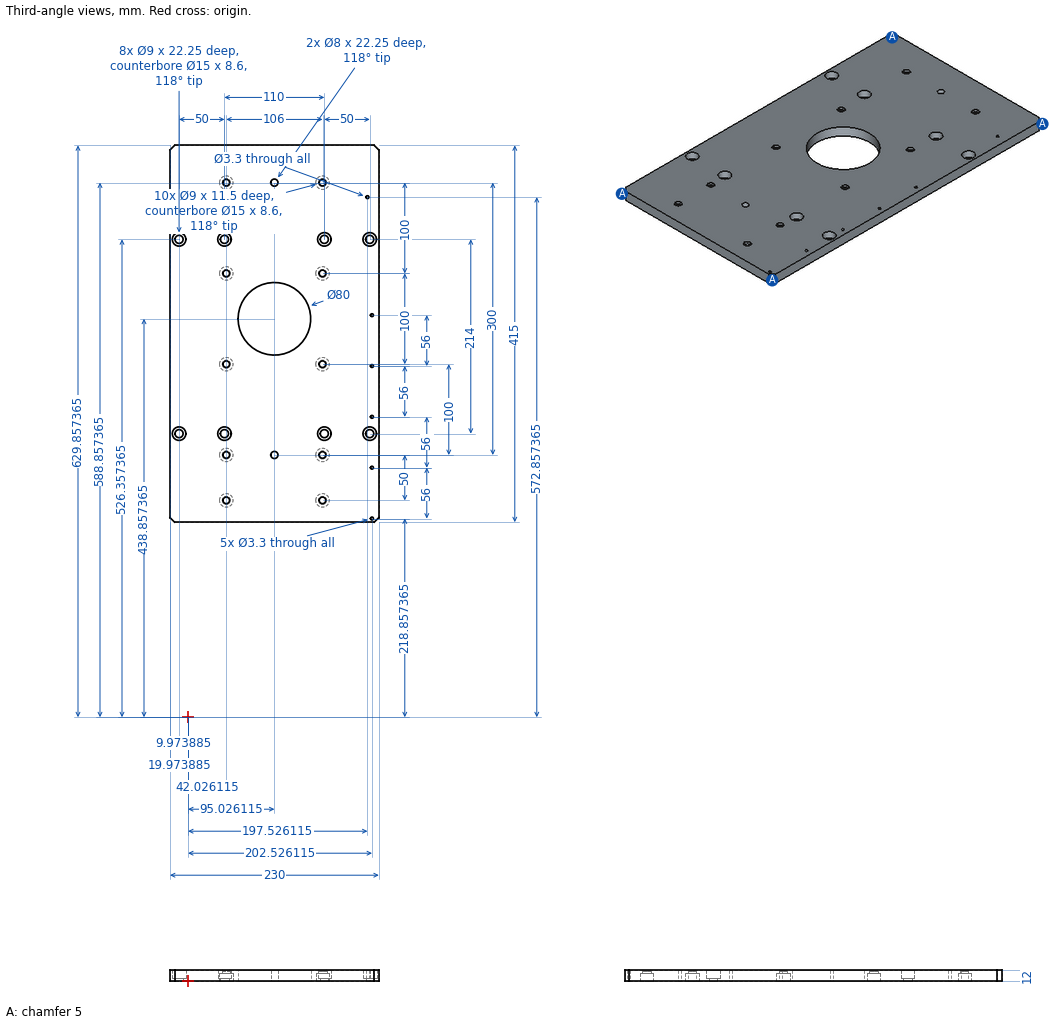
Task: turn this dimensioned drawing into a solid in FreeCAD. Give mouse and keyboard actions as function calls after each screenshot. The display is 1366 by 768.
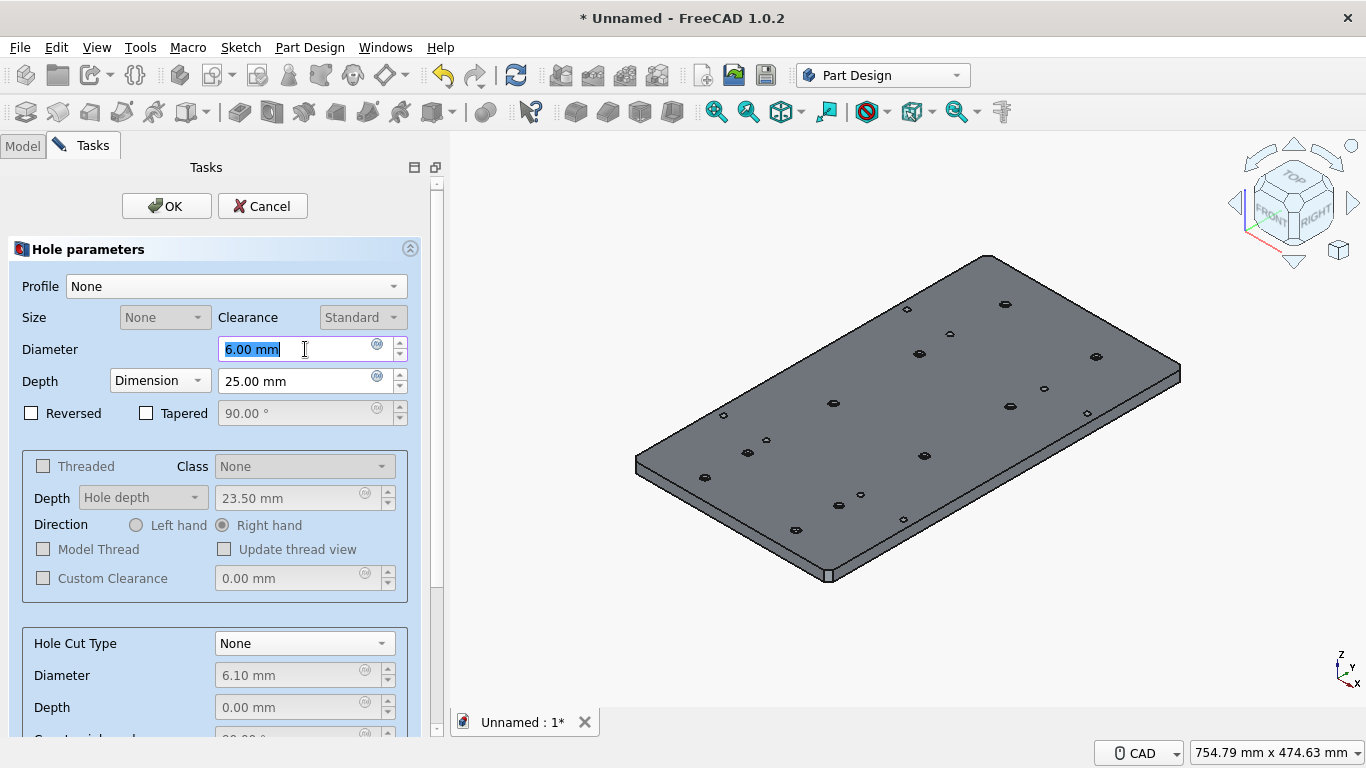
text(9)
key(Tab)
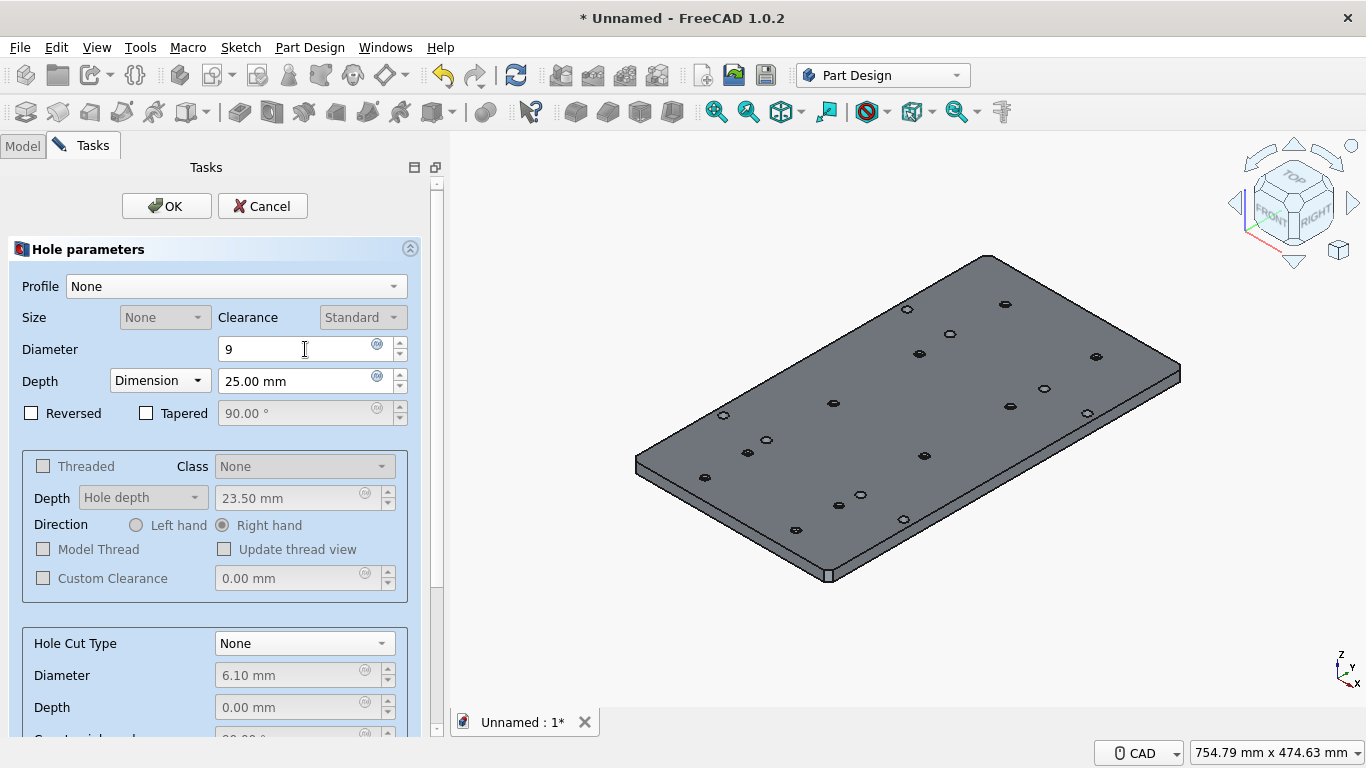
triple_click(305, 381)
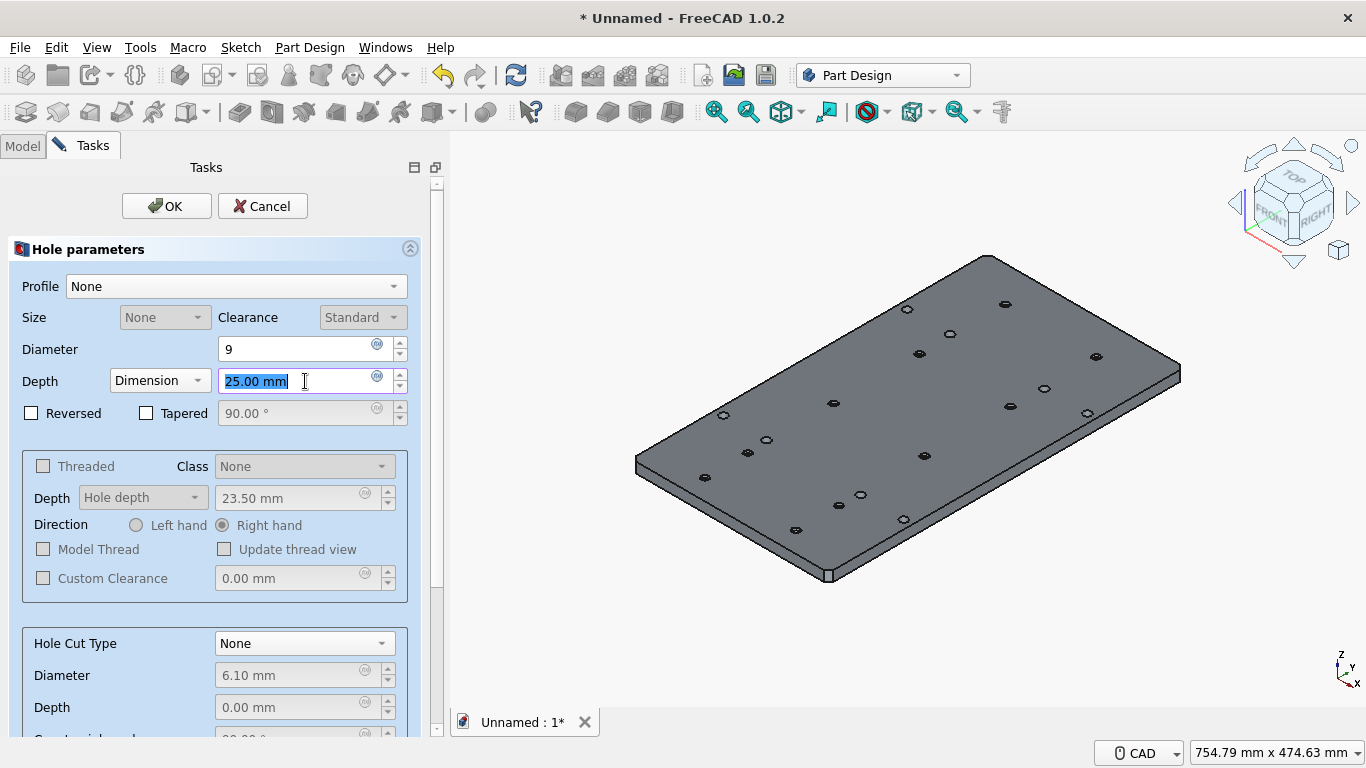
text(22.25)
key(Tab)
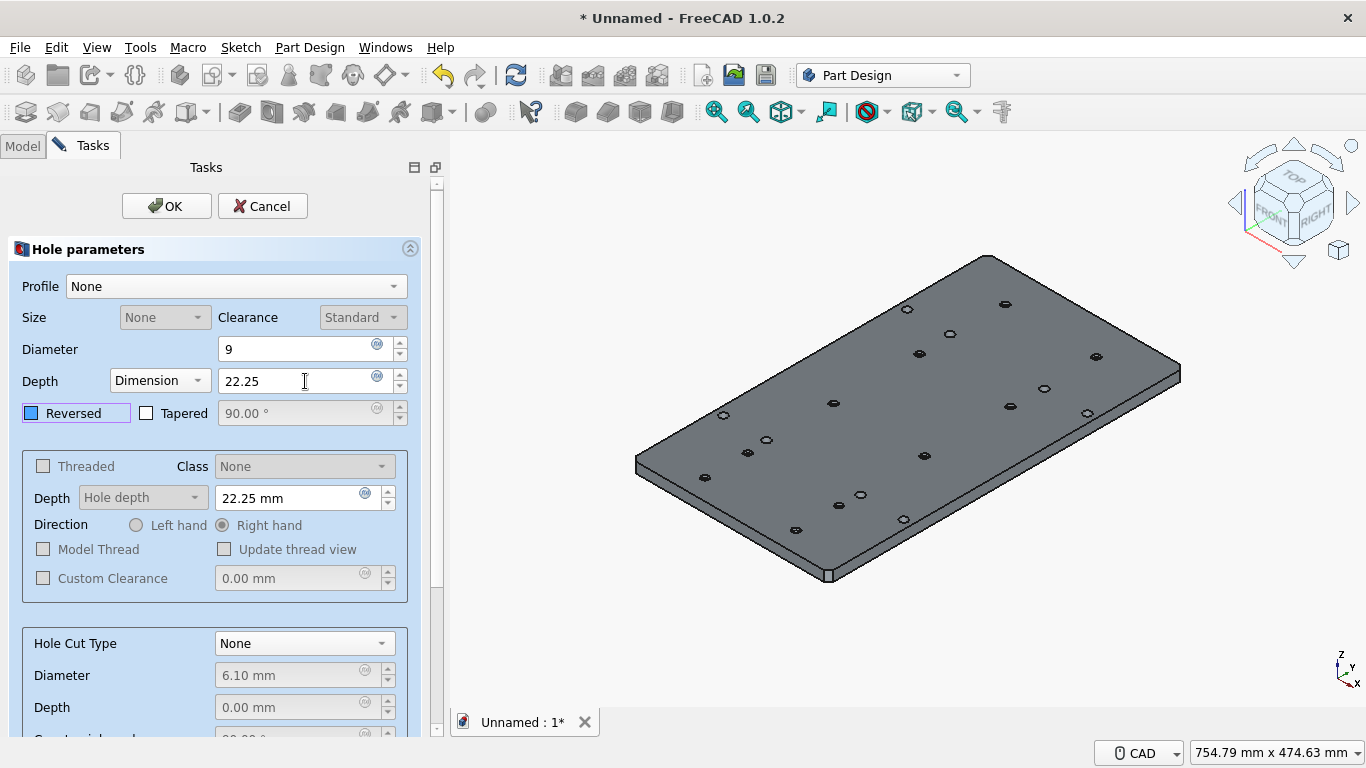
click(306, 644)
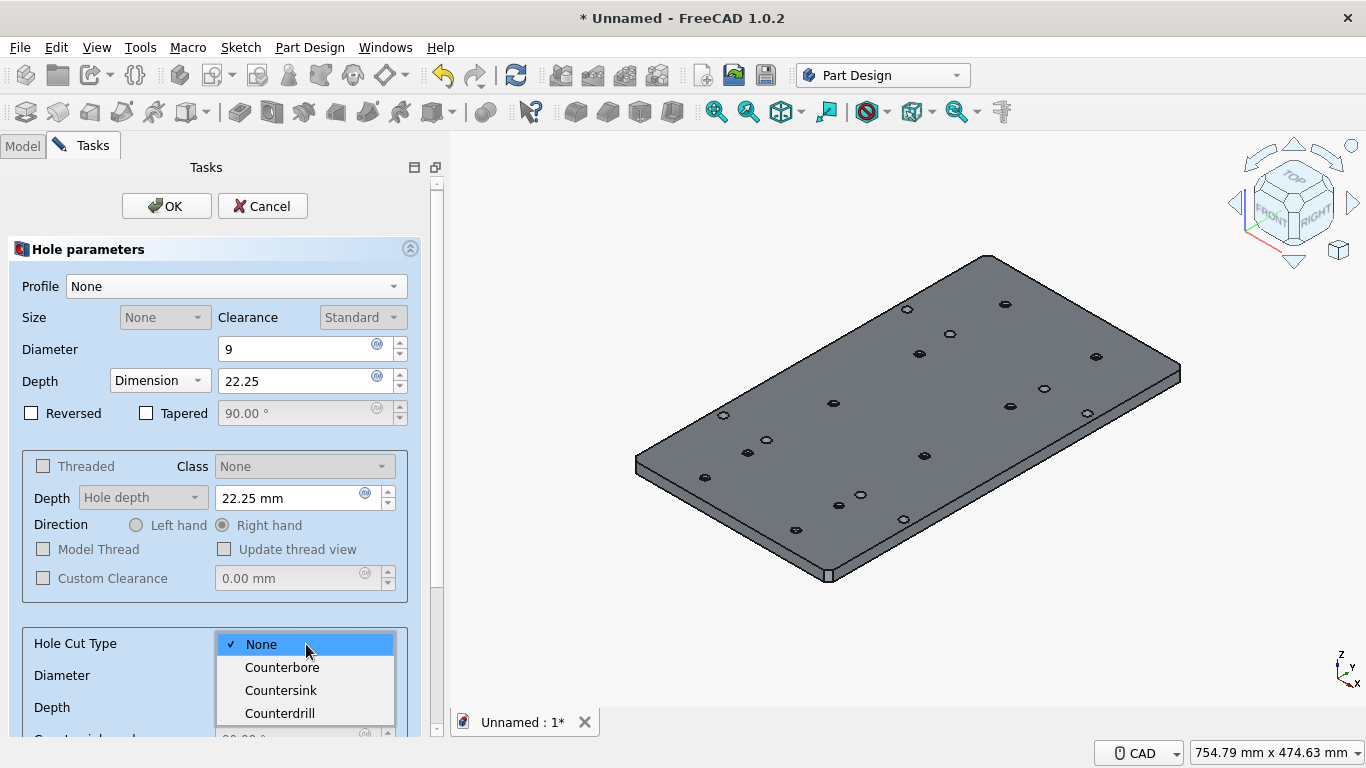
click(304, 668)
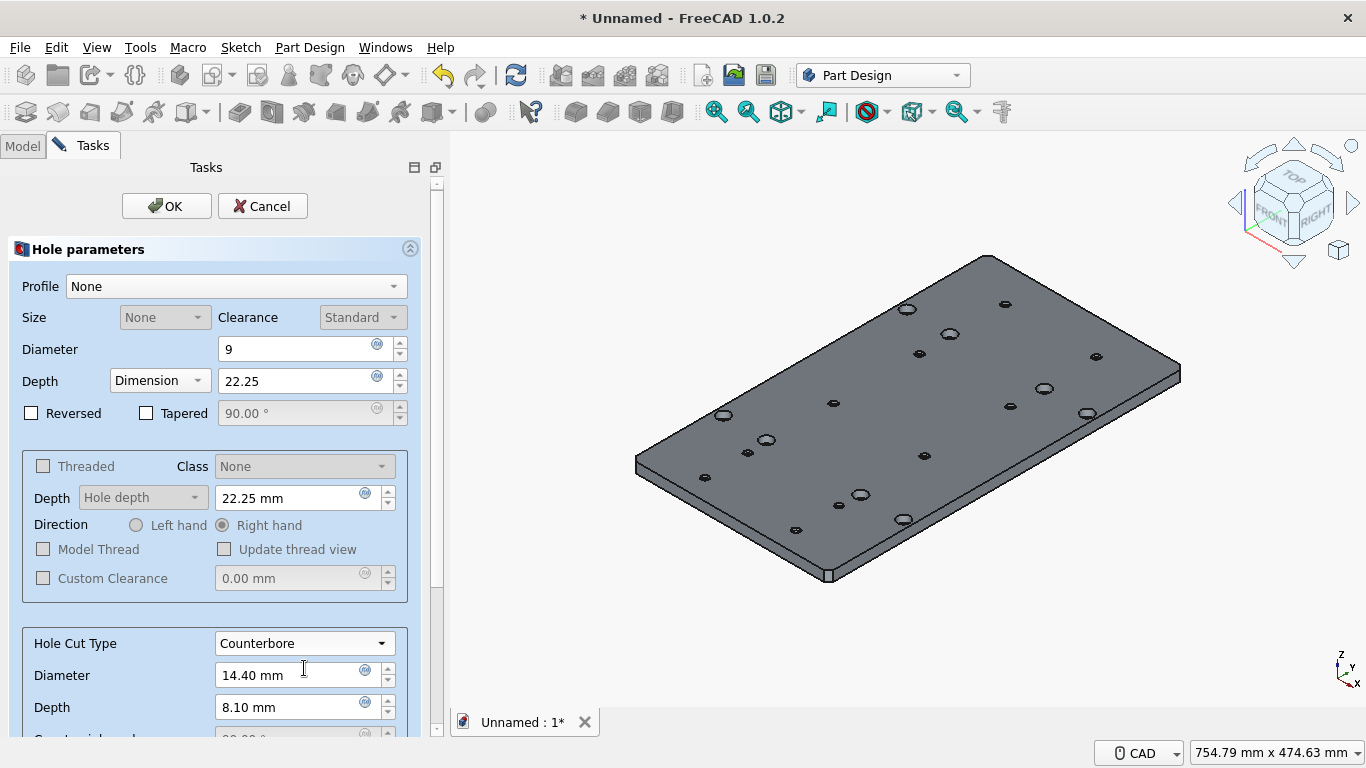
triple_click(298, 675)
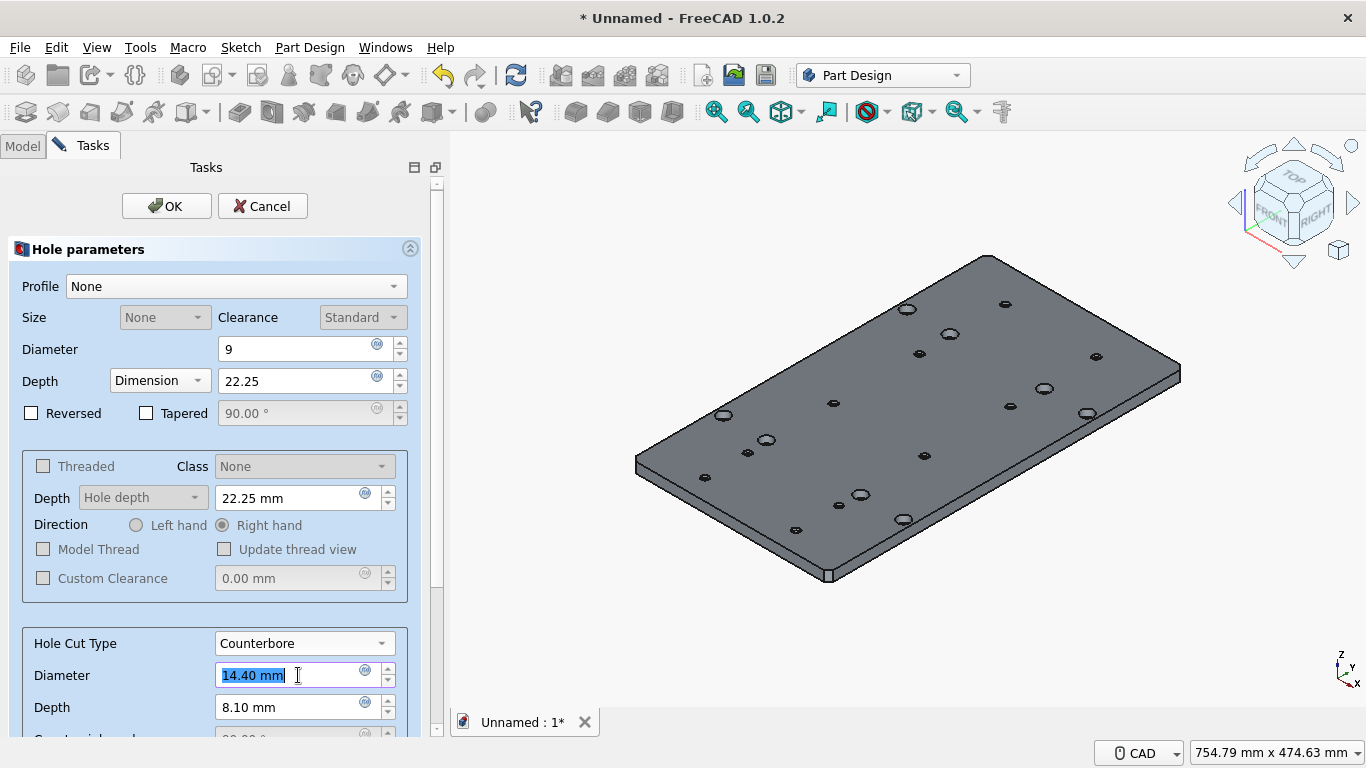
text(15)
key(Tab)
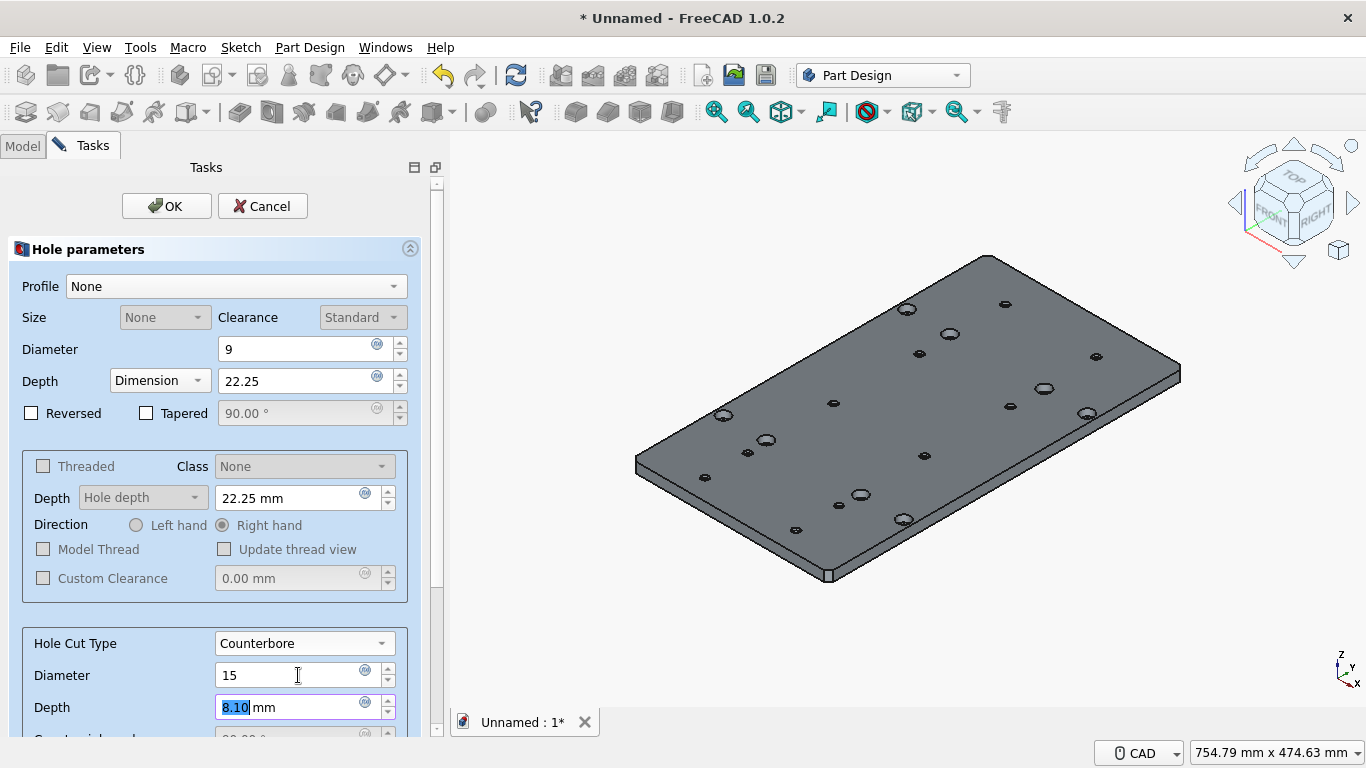
text(8.6)
key(Tab)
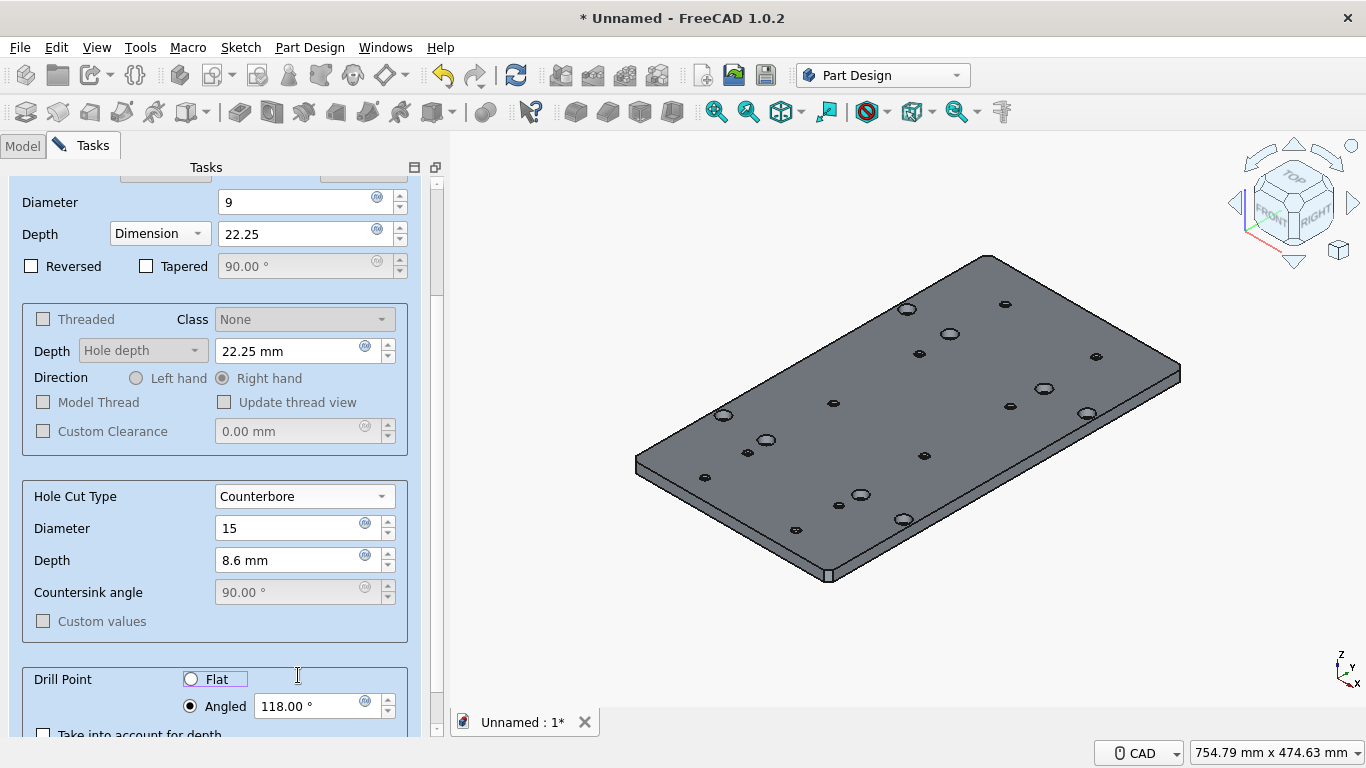
scroll(437, 456, up, 4)